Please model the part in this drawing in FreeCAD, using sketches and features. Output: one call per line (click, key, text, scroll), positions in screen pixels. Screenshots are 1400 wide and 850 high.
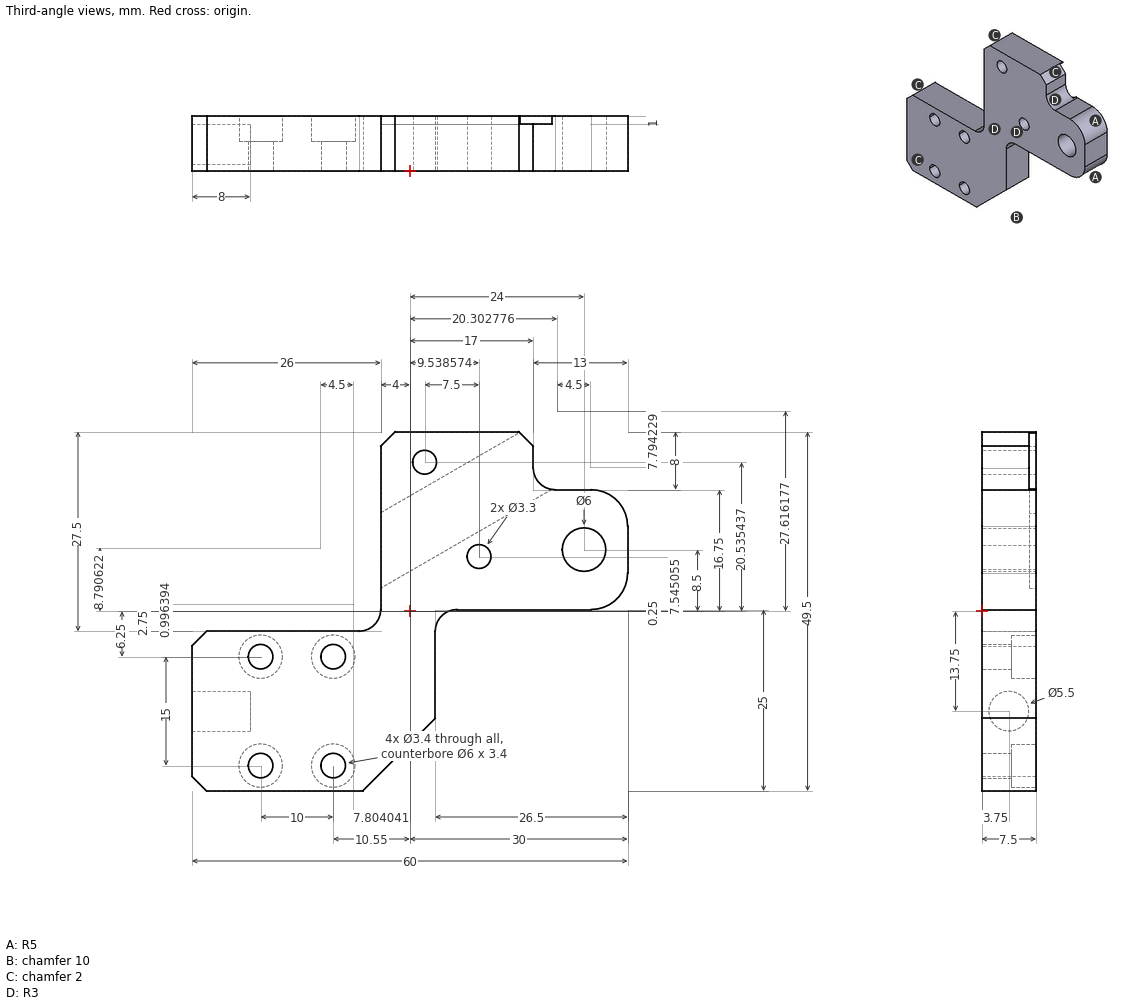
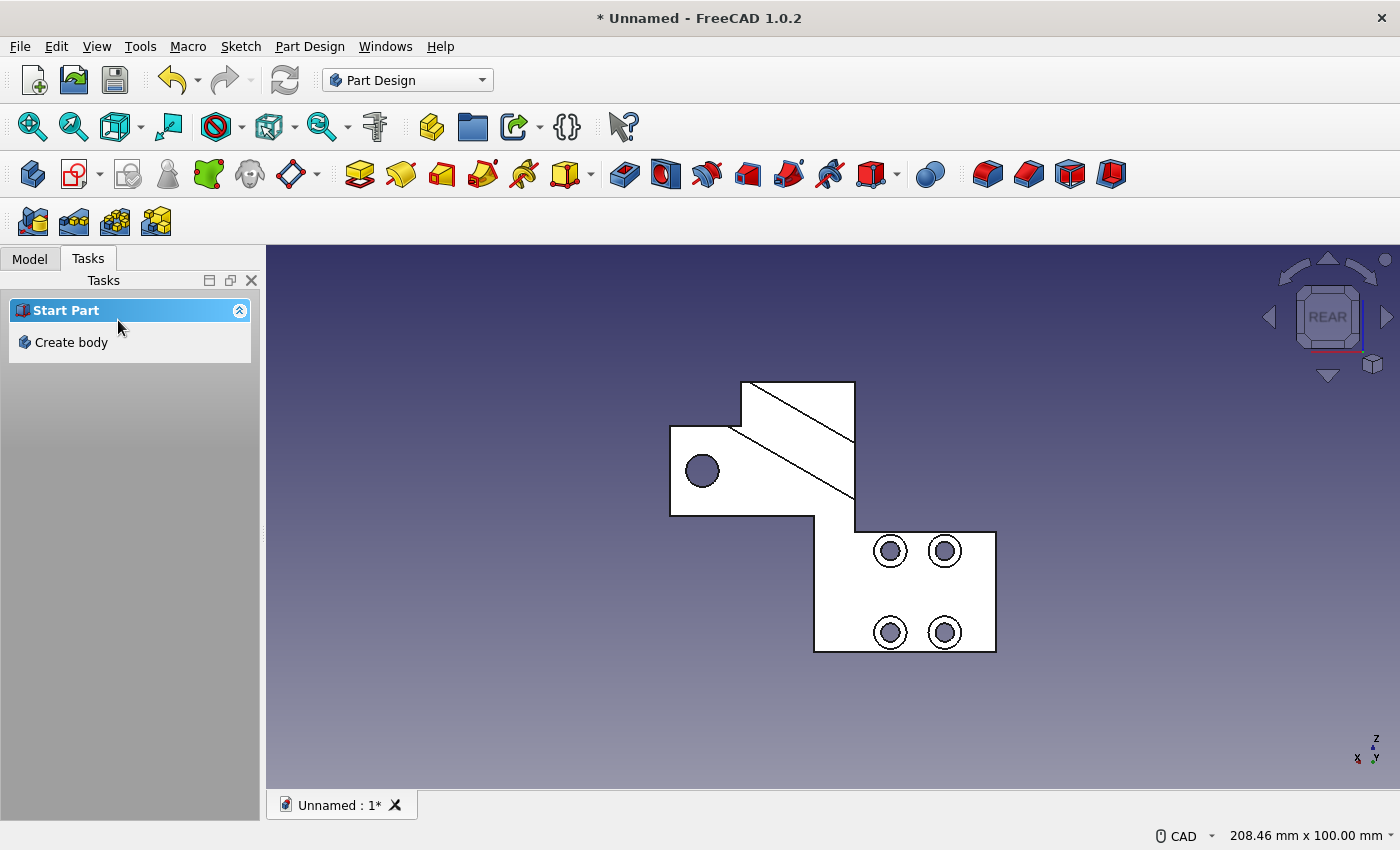
key(0)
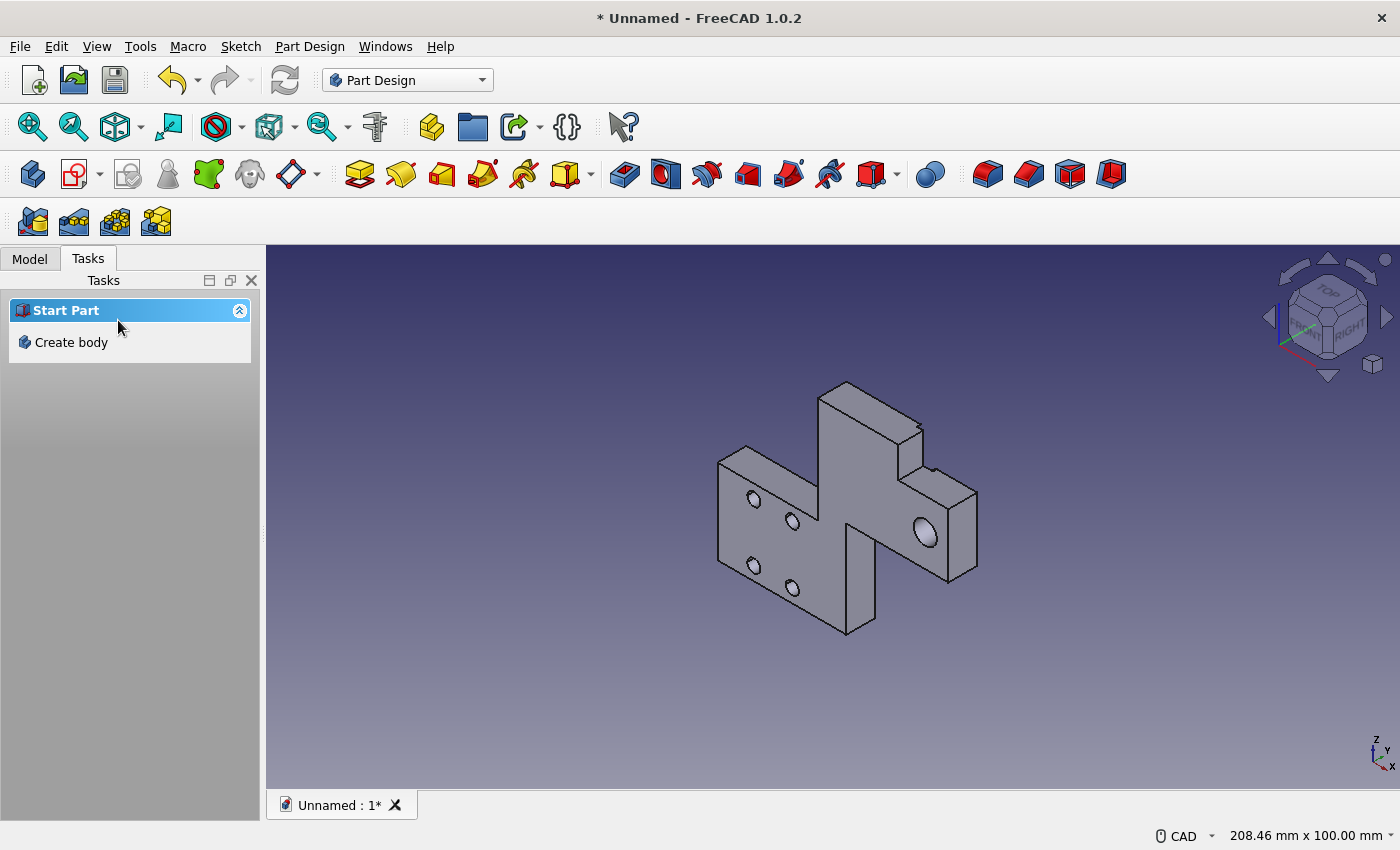
click(963, 500)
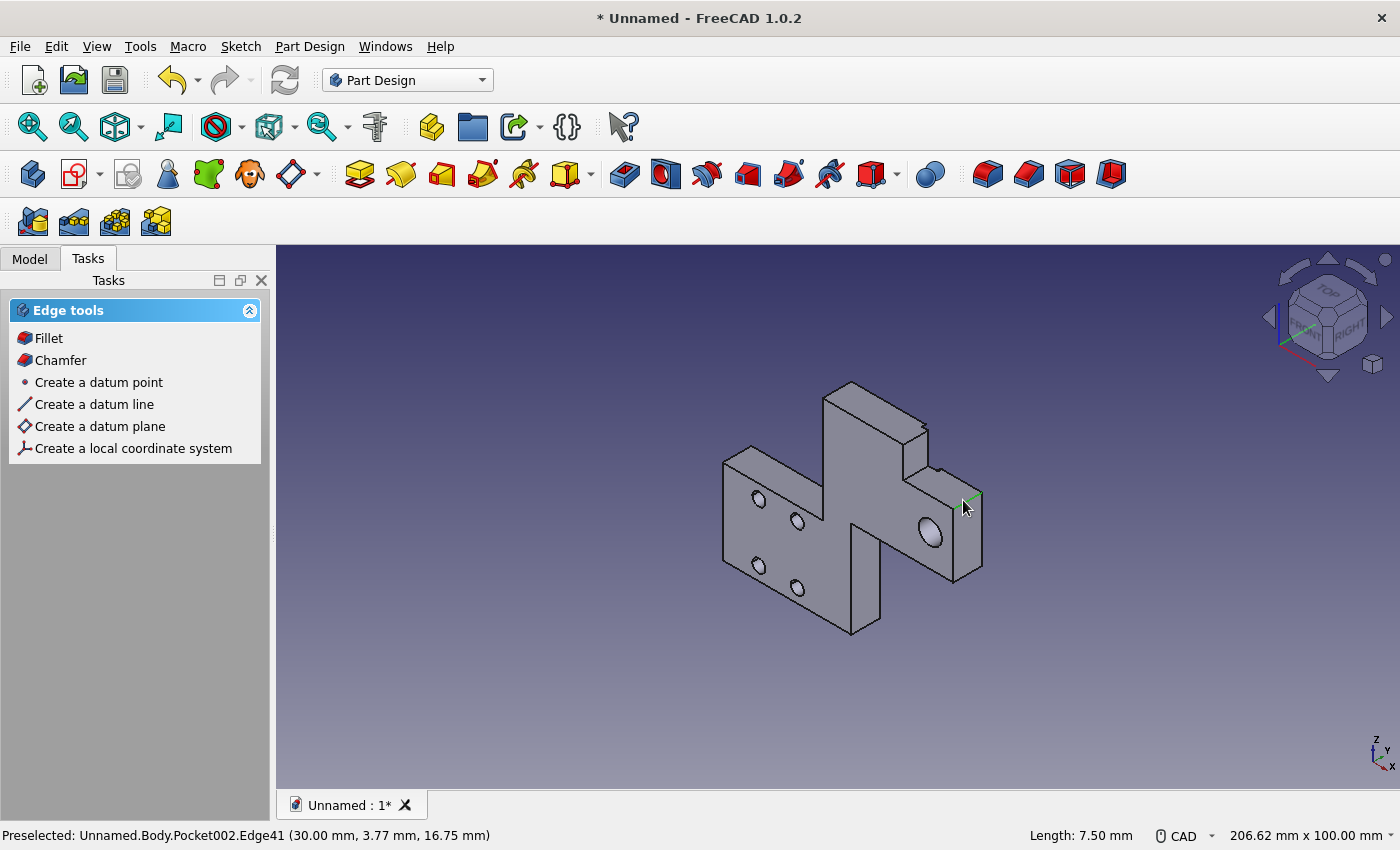
key(2)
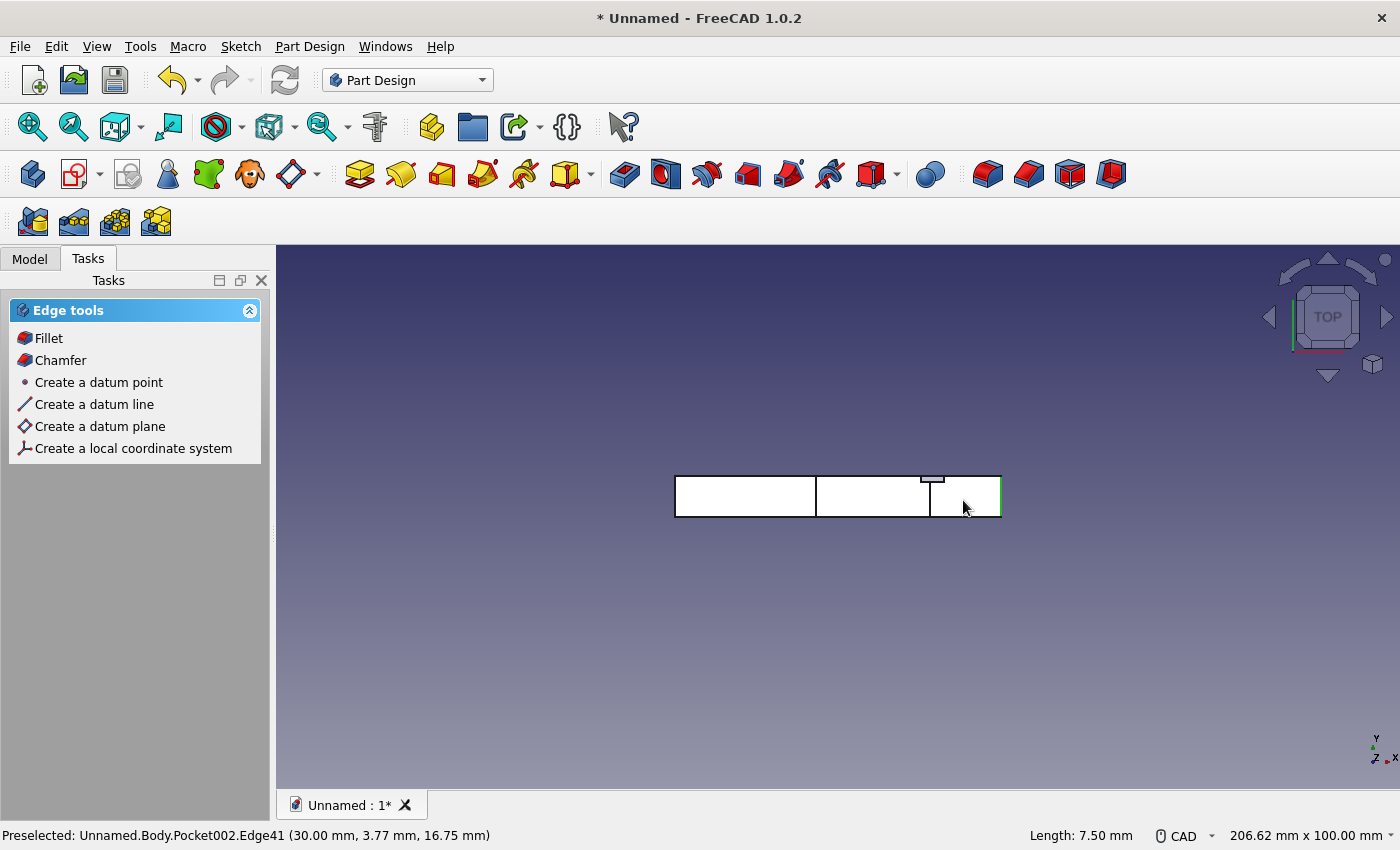
key(v)
key(f)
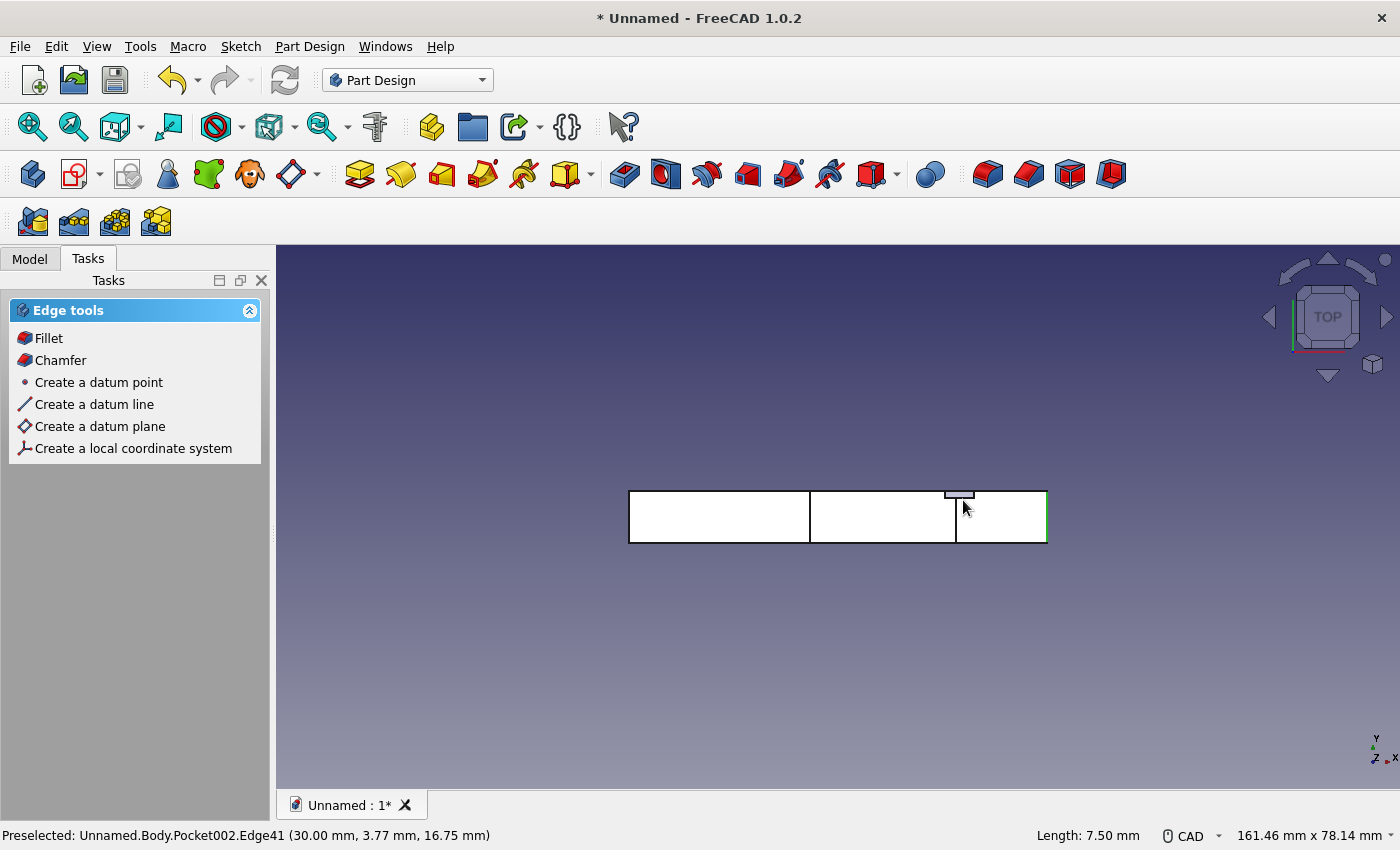
key(1)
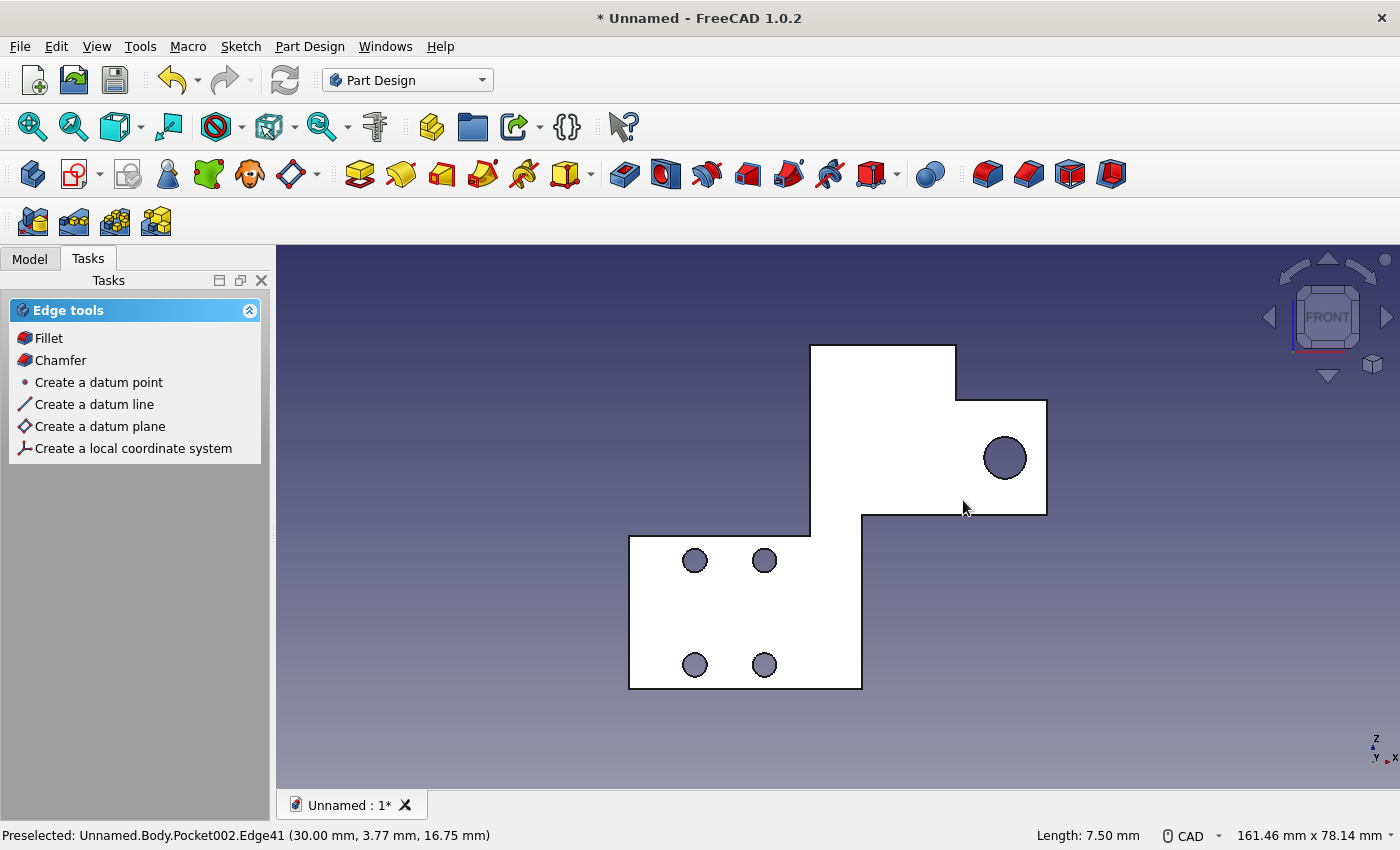
key(3)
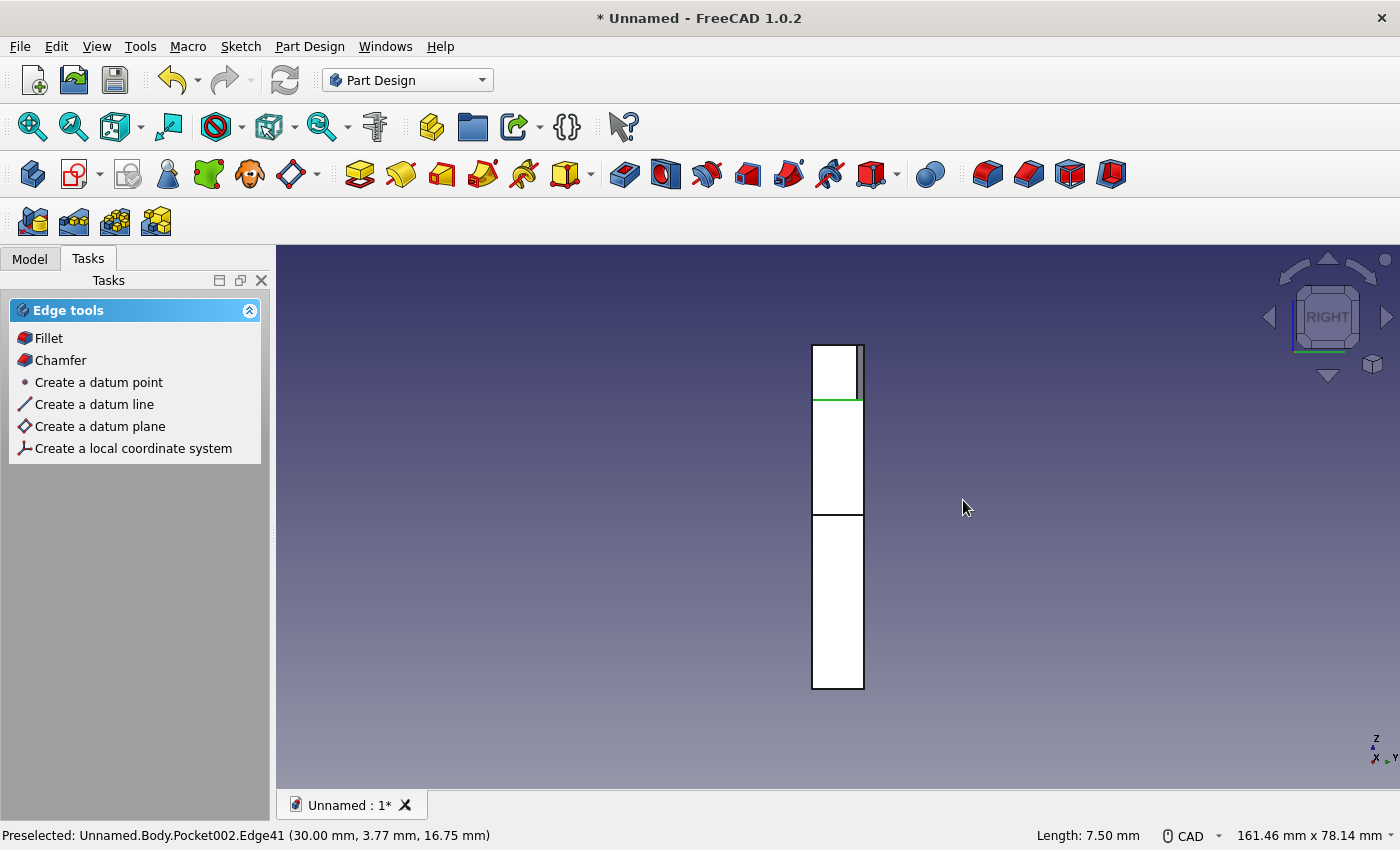
click(838, 514, ctrl)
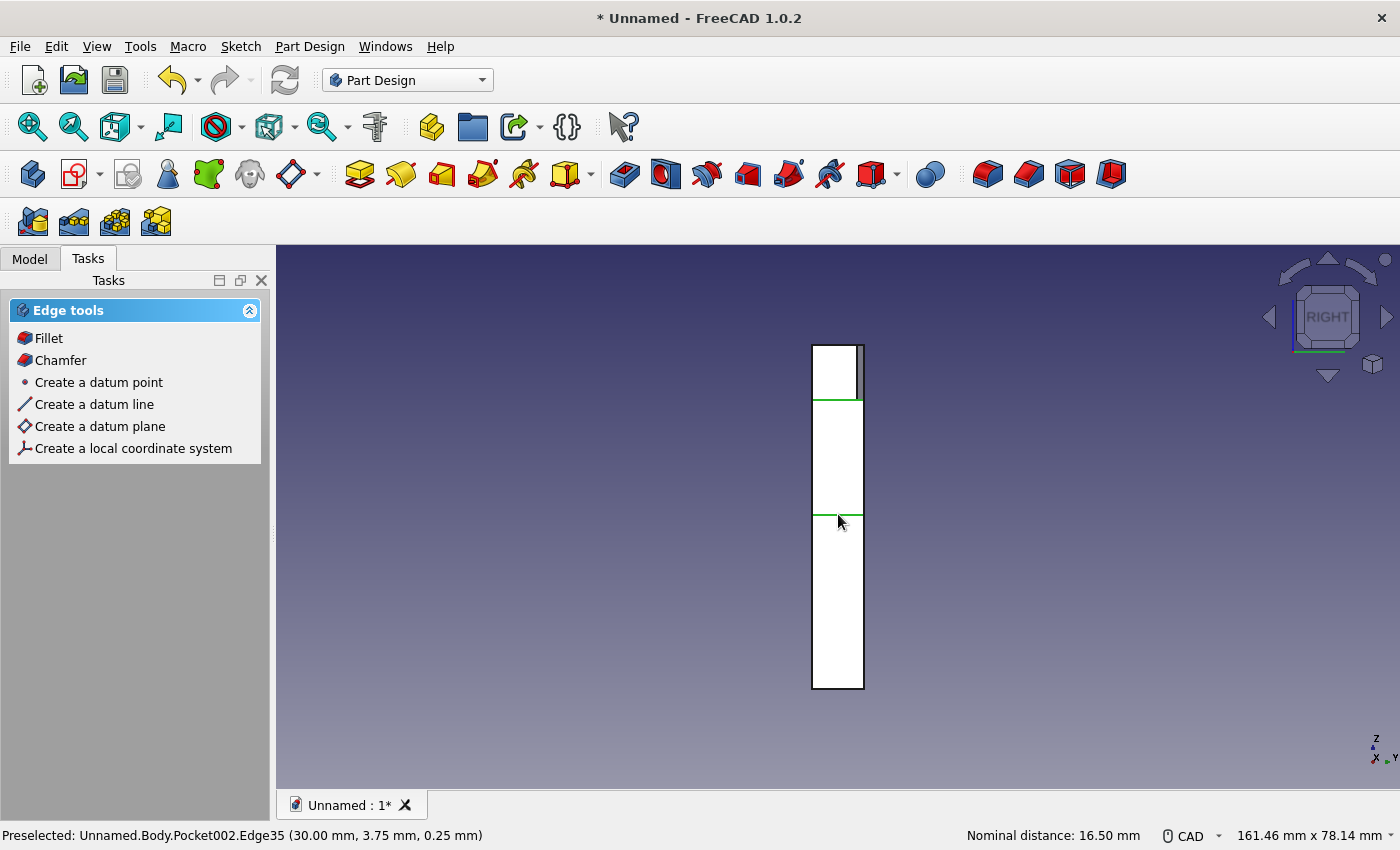
click(988, 174)